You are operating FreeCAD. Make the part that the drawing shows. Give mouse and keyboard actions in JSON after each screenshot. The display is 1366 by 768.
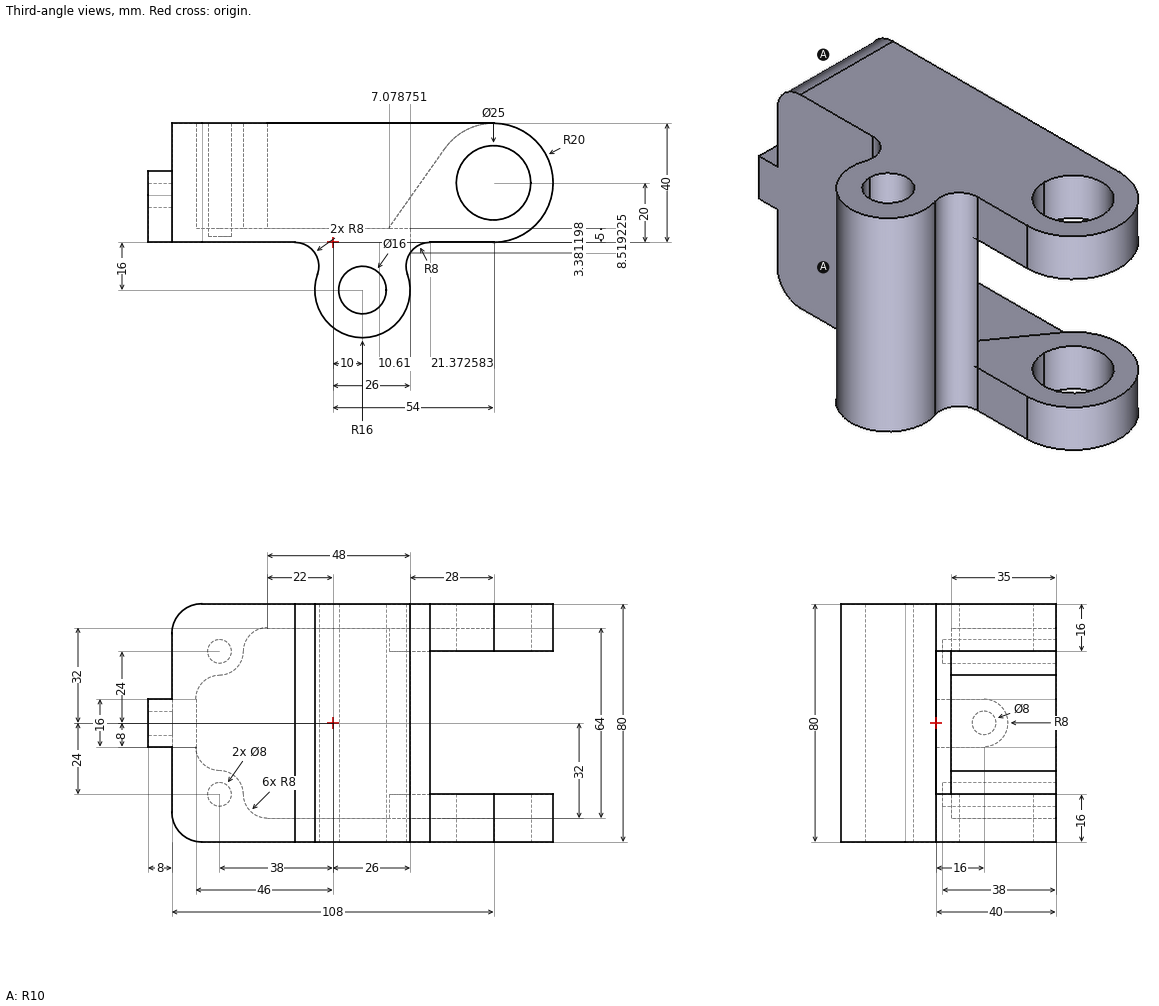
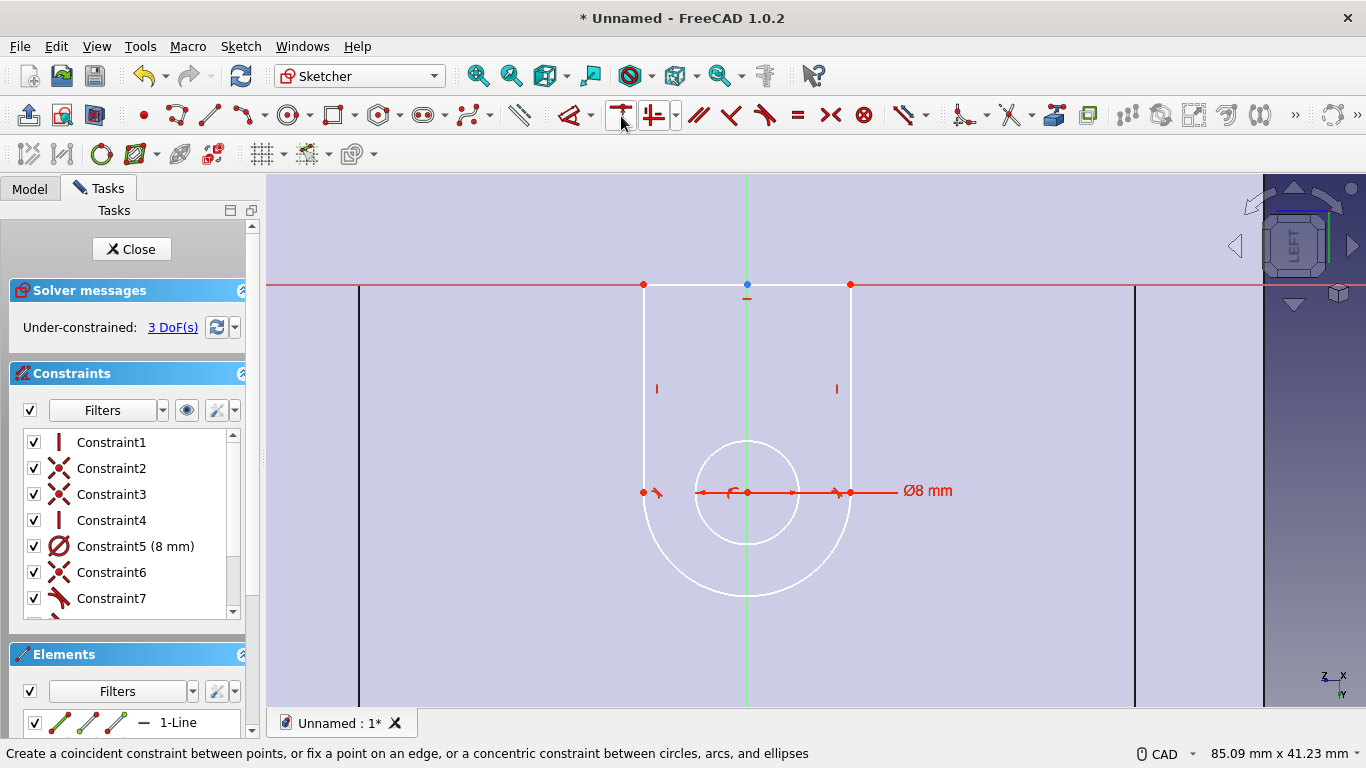
{"action": "left_click", "coordinate": [568, 116]}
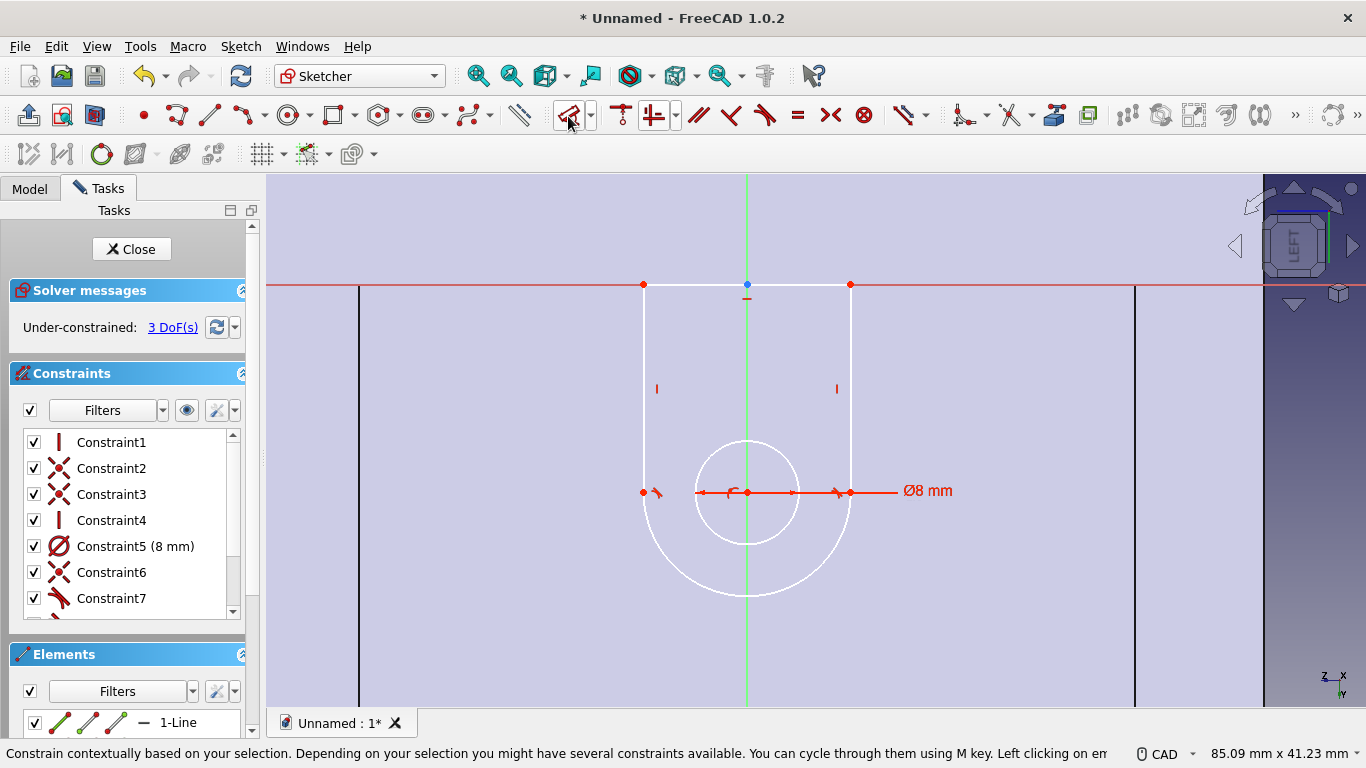
{"action": "left_click", "coordinate": [686, 576]}
{"action": "left_click", "coordinate": [667, 602]}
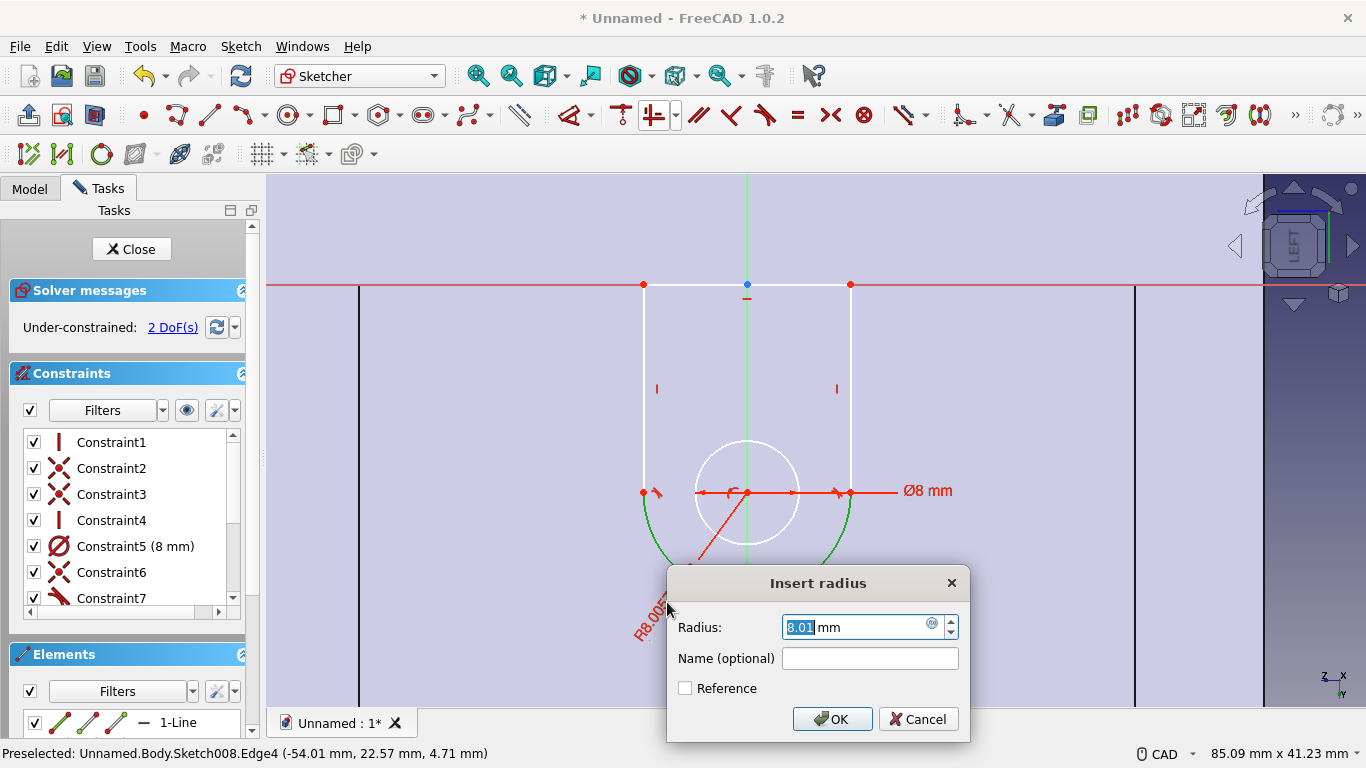
{"action": "type", "text": "8"}
{"action": "key", "text": "Return"}
{"action": "key", "text": "Escape"}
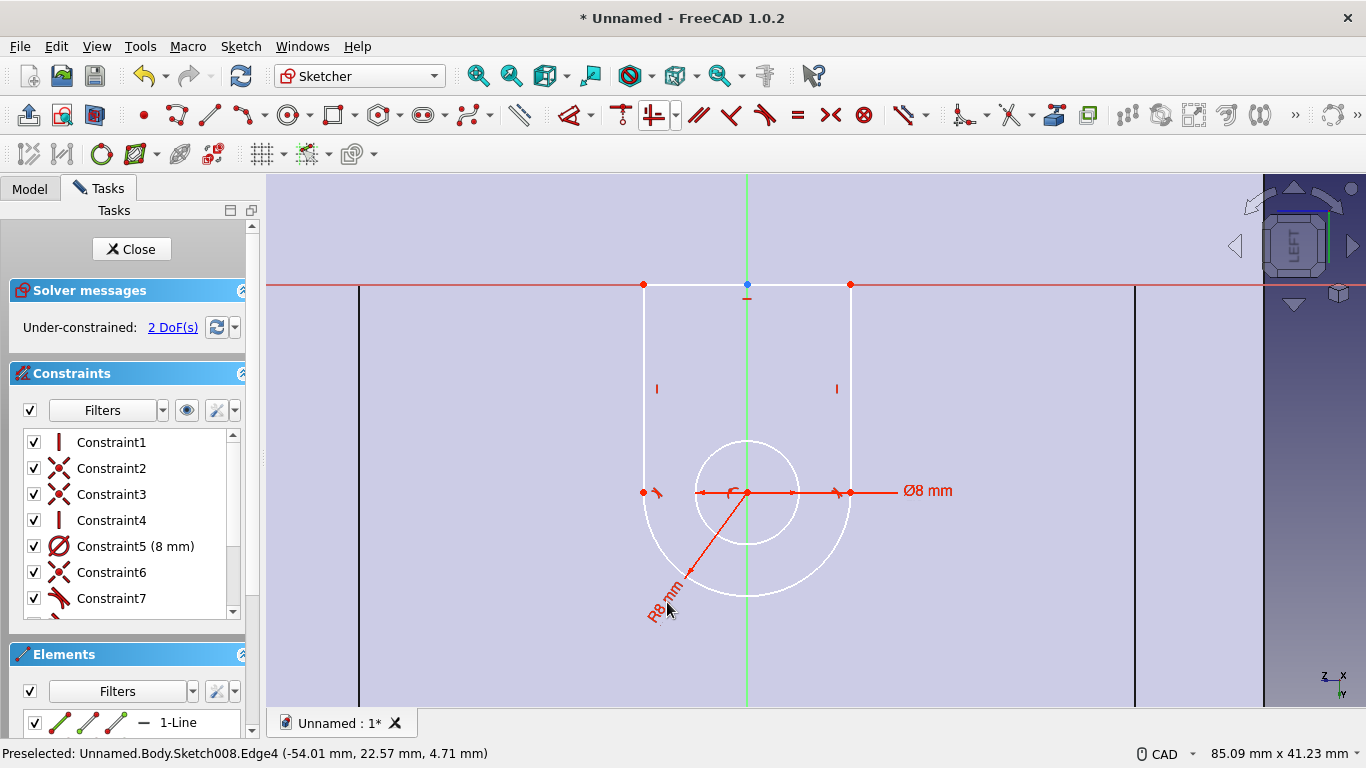
{"action": "left_click", "coordinate": [851, 285]}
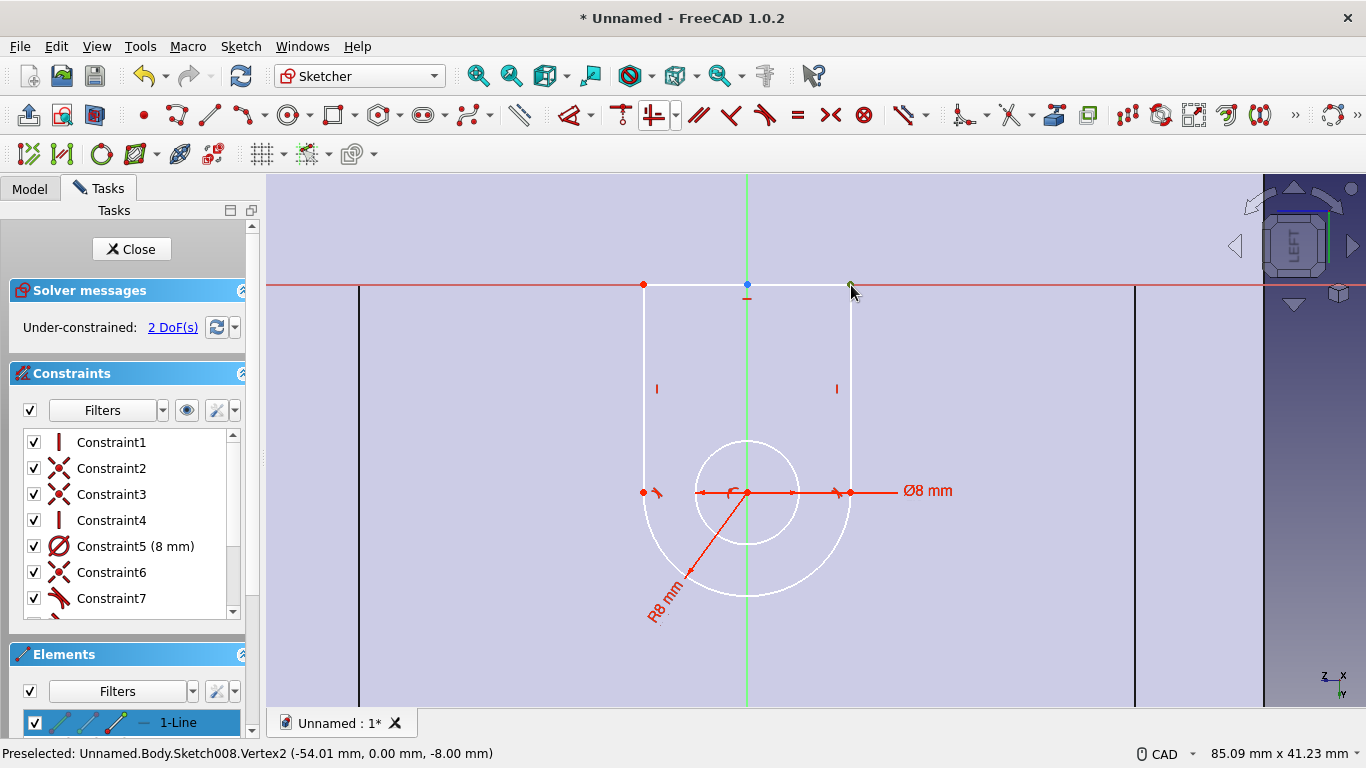
{"action": "left_click", "coordinate": [359, 285]}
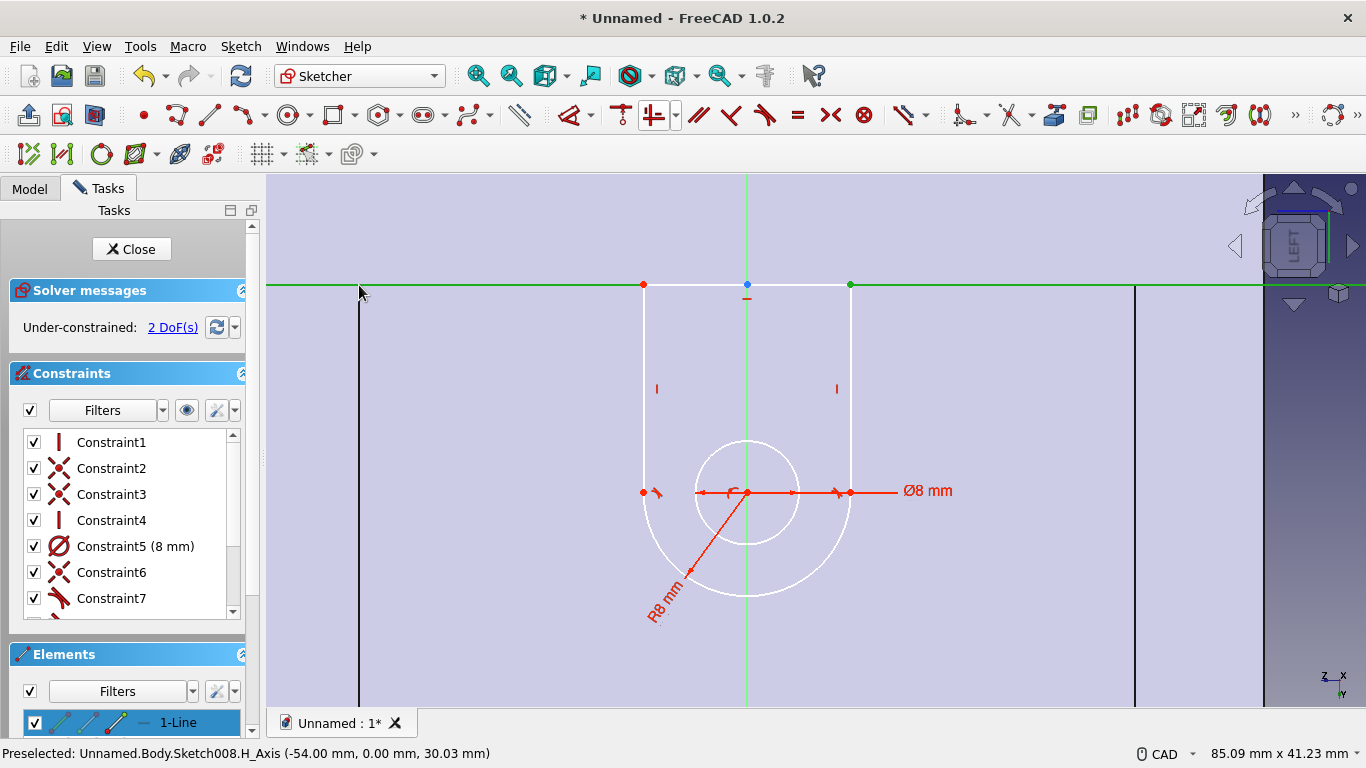
{"action": "key", "text": "c"}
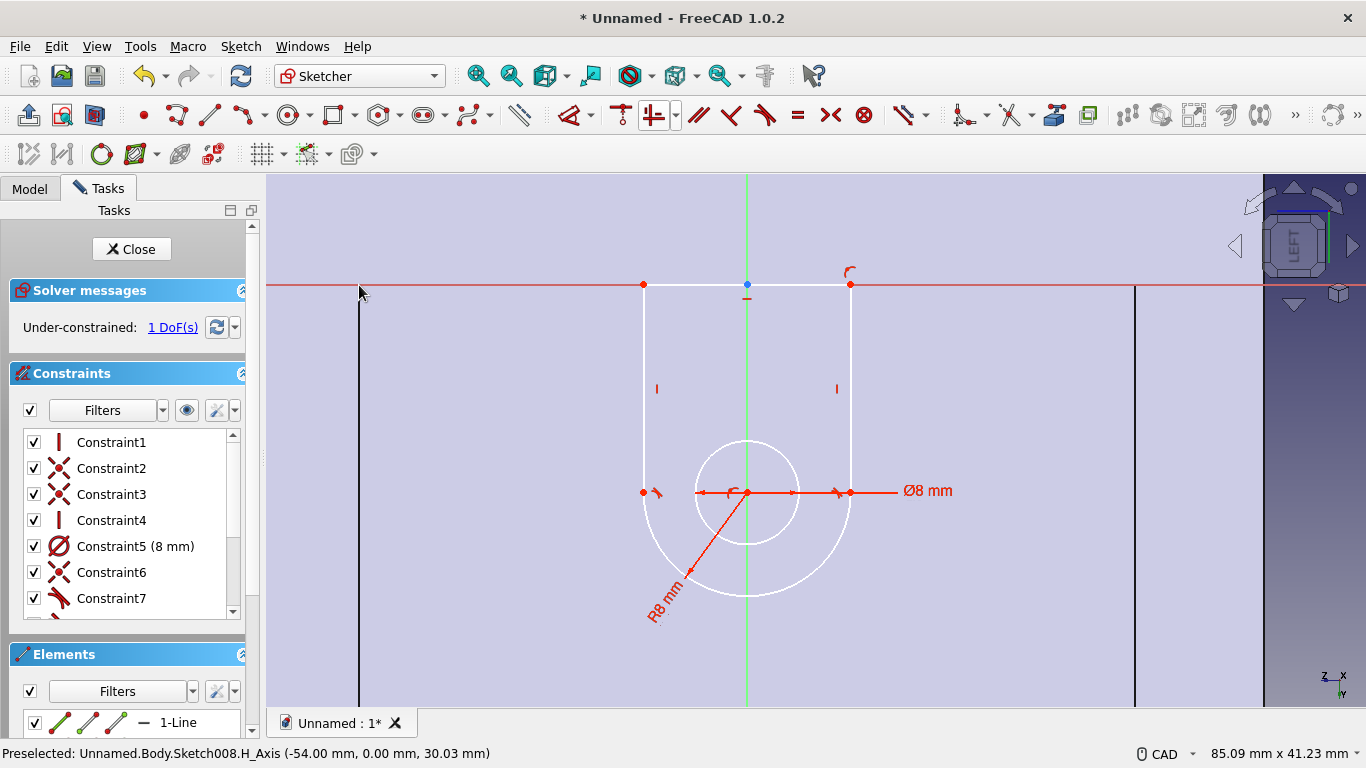
{"action": "key", "text": "d"}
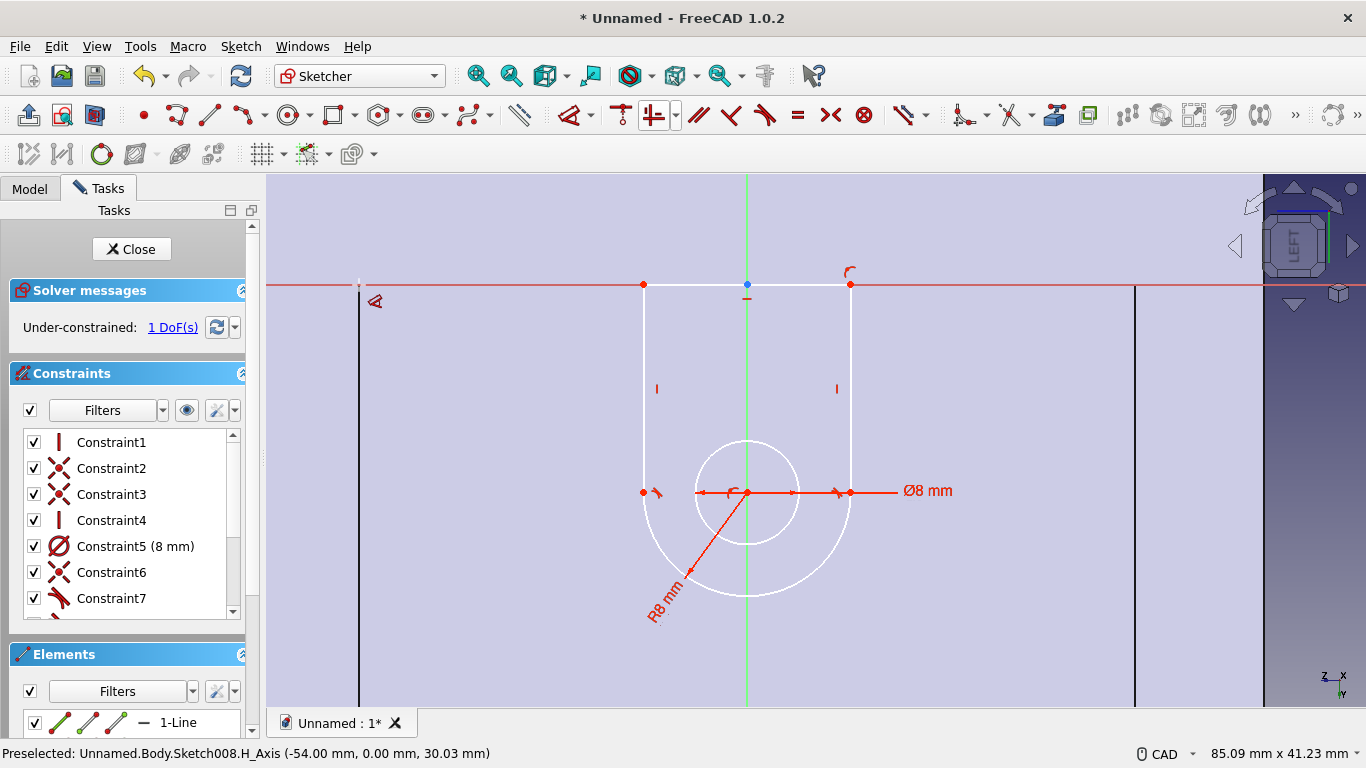
{"action": "left_click", "coordinate": [851, 430]}
{"action": "left_click", "coordinate": [885, 389]}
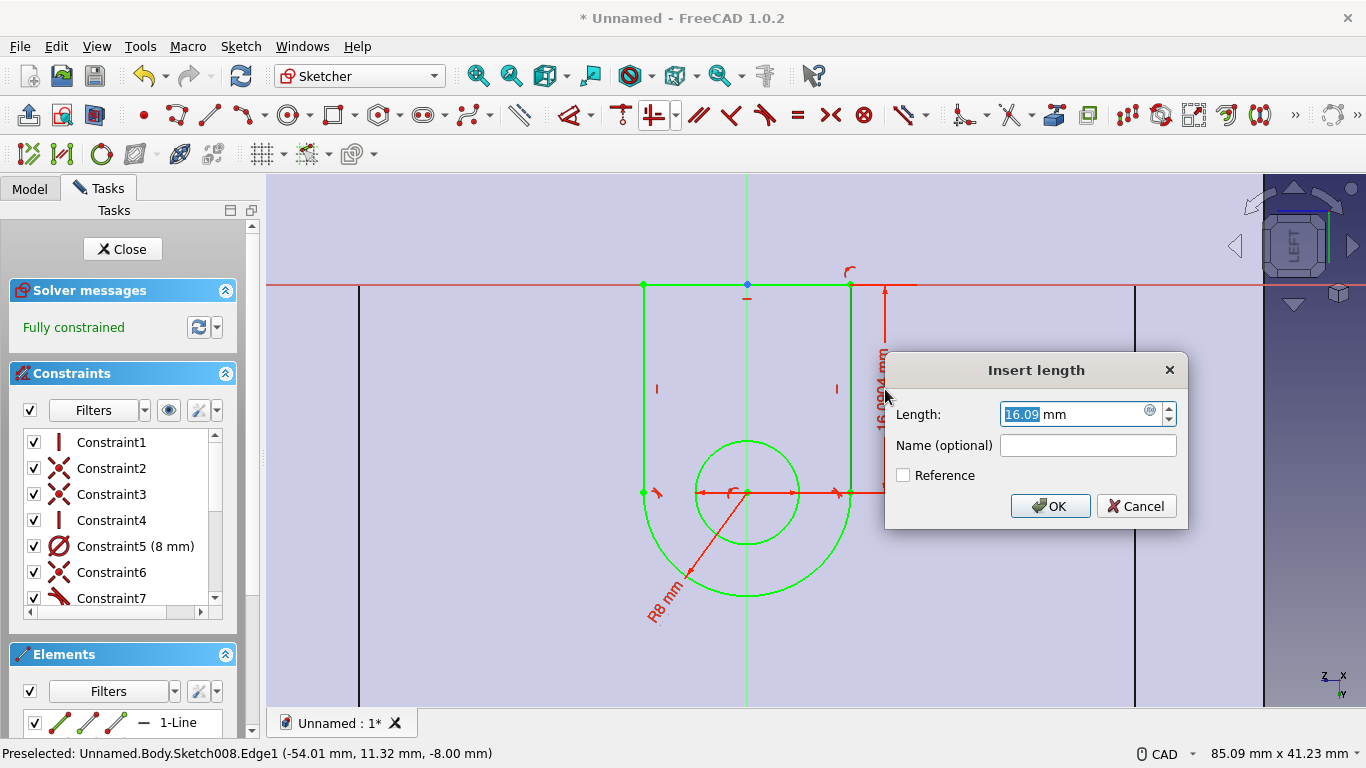
{"action": "type", "text": "16"}
{"action": "key", "text": "Return"}
{"action": "key", "text": "Escape"}